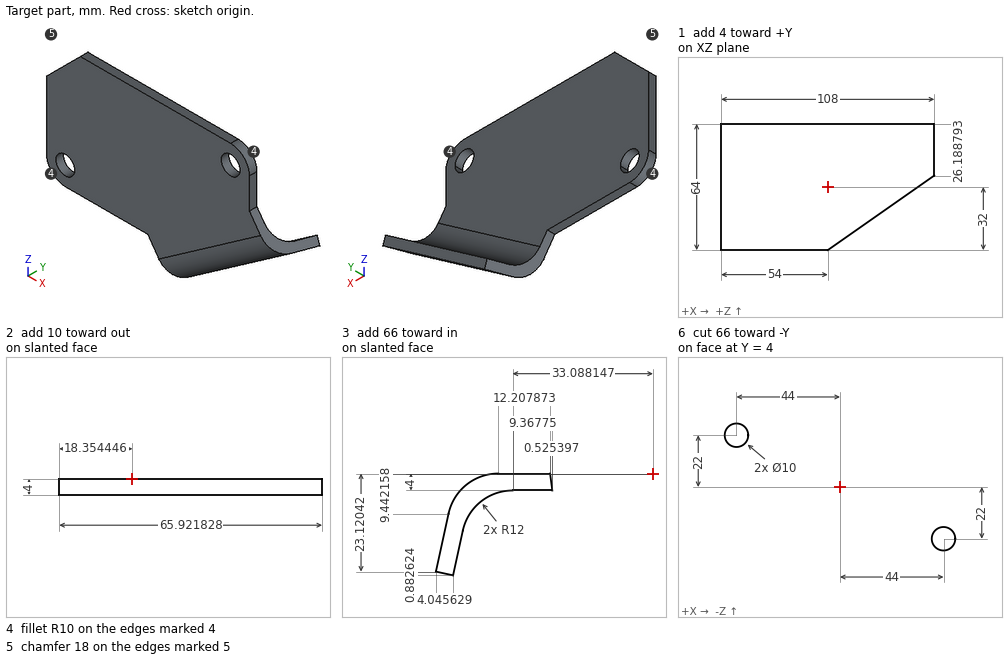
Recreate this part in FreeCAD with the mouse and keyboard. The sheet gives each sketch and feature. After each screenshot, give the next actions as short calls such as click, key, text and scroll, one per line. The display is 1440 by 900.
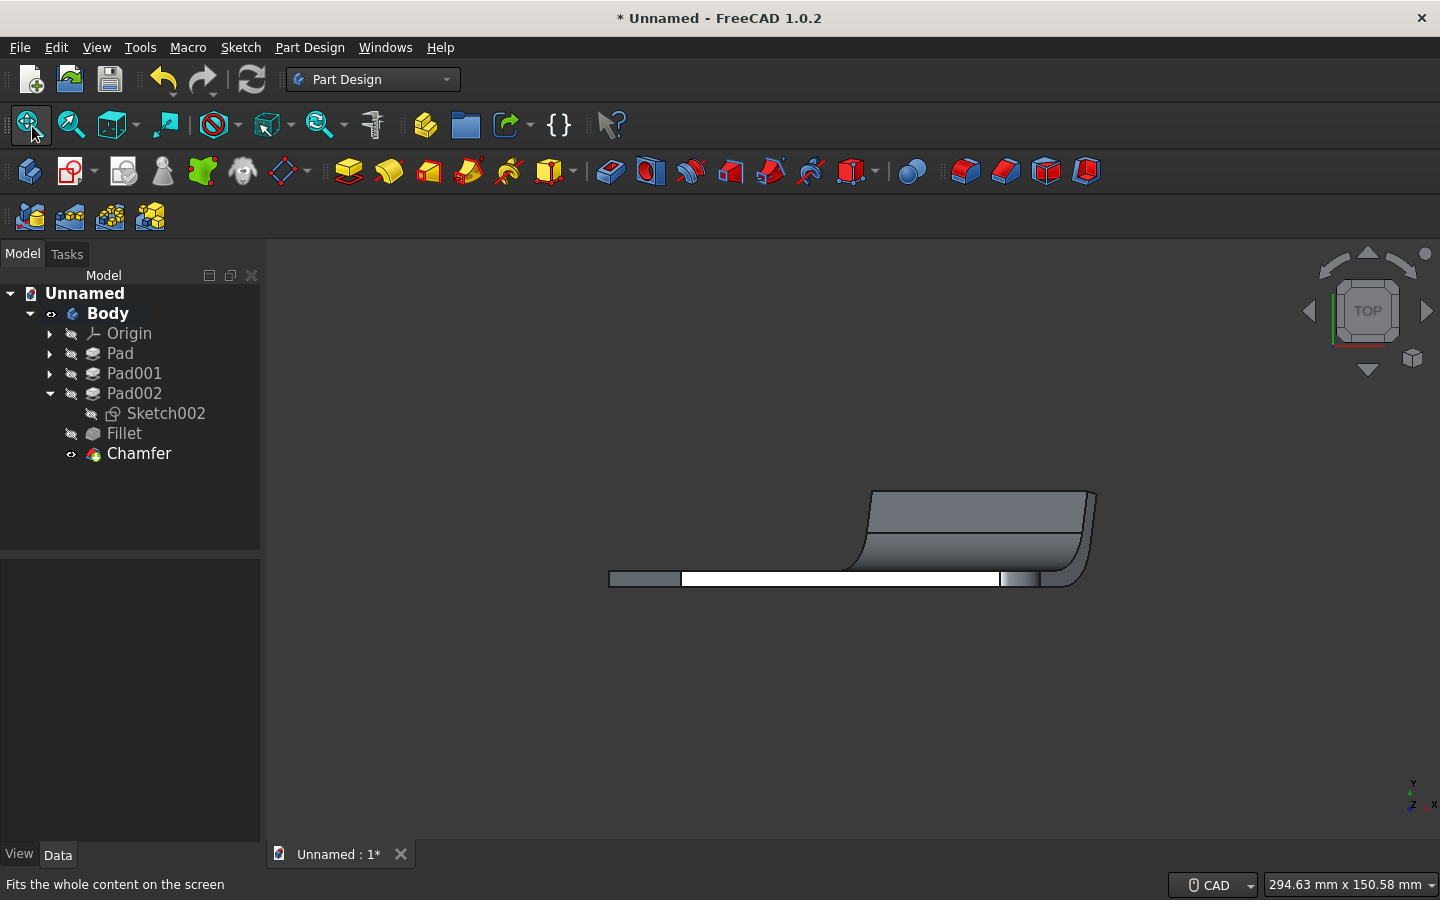
key(4)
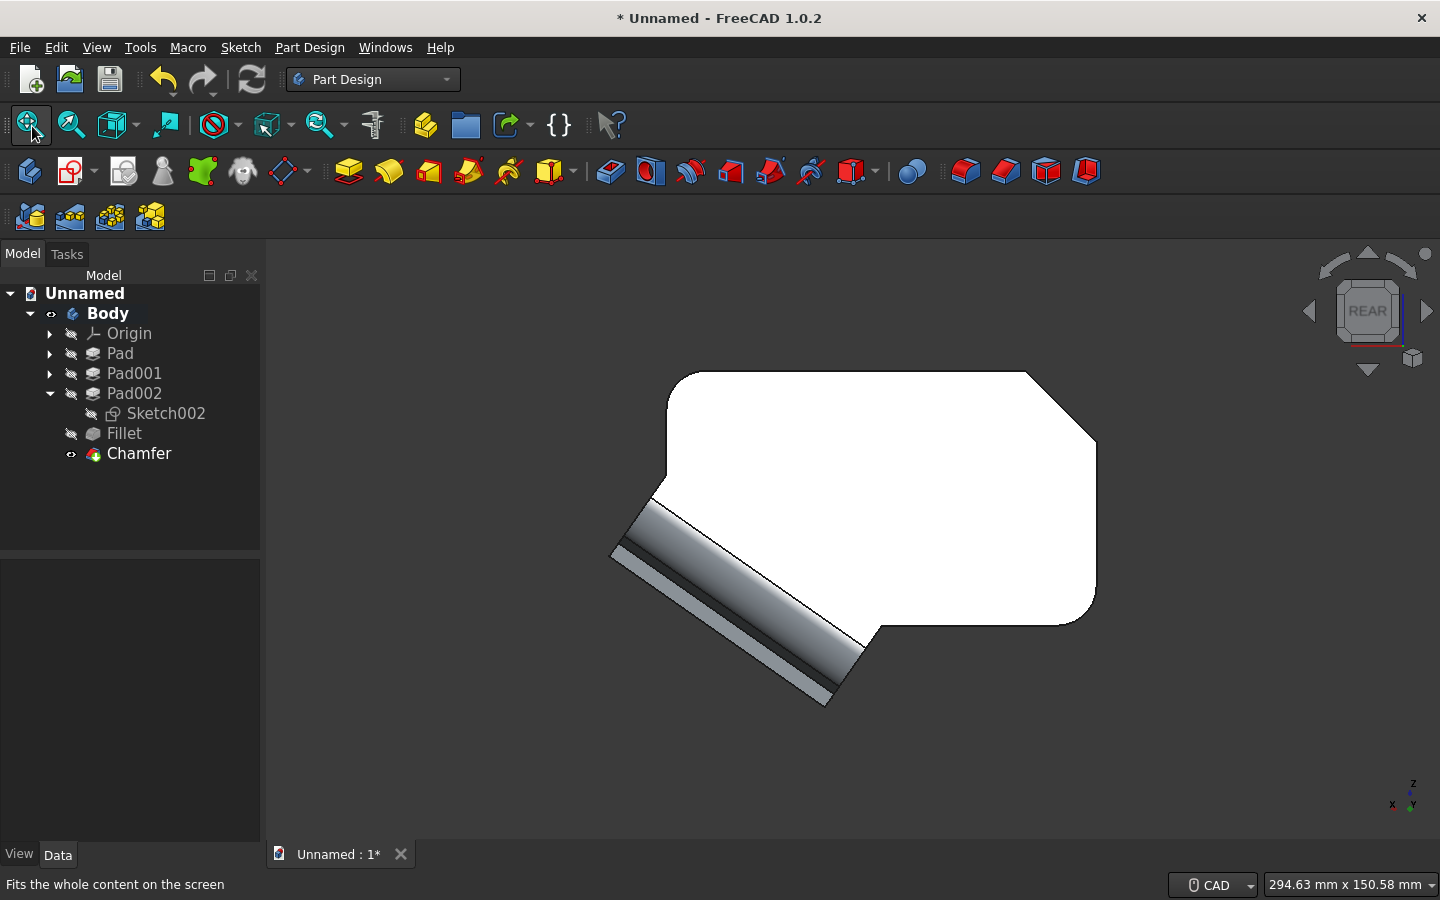
click(874, 509)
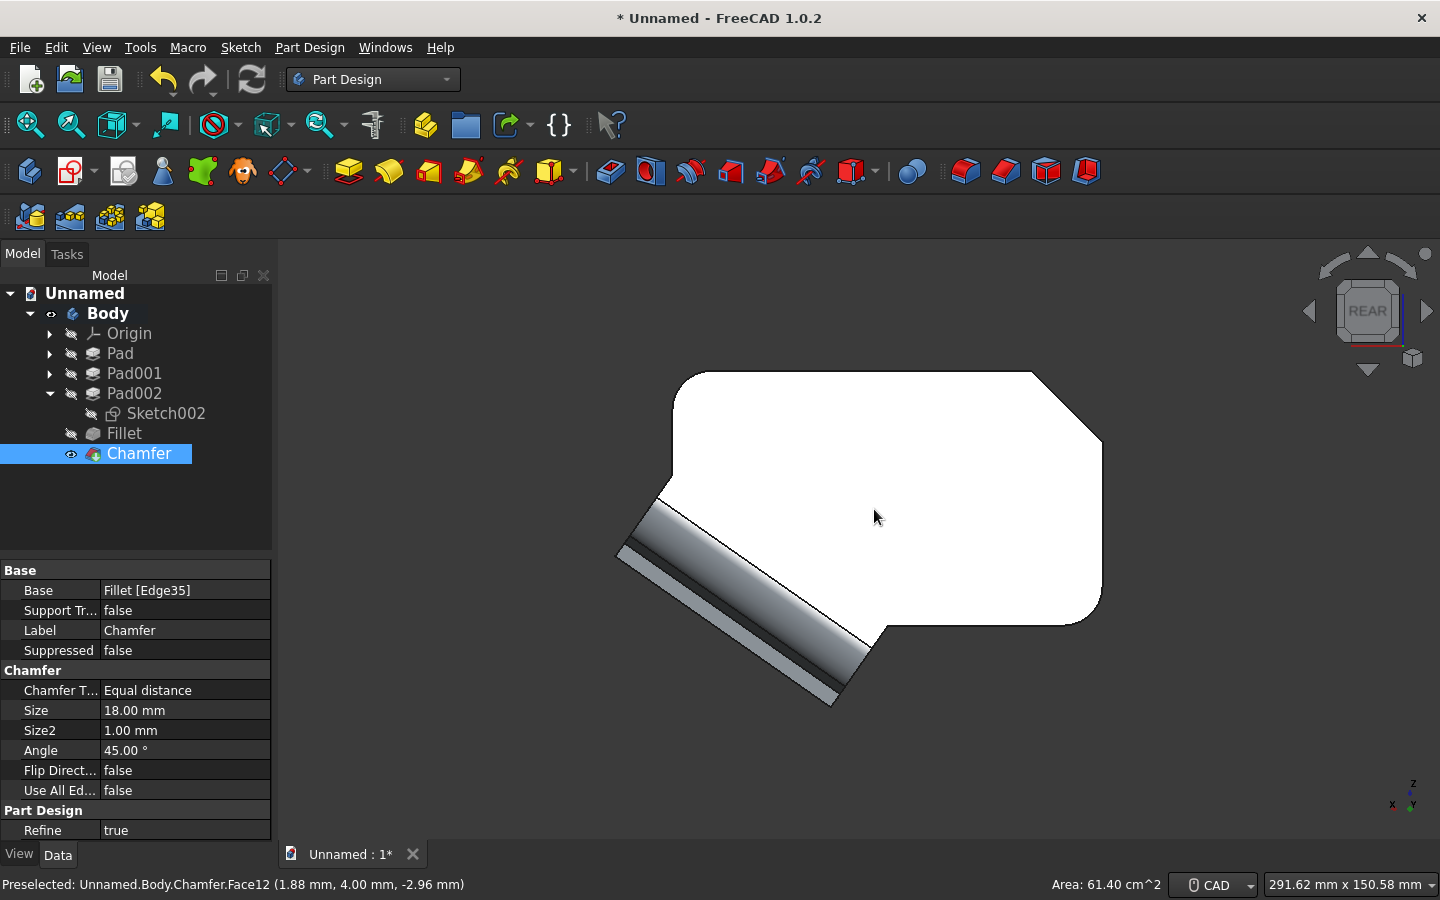
click(70, 172)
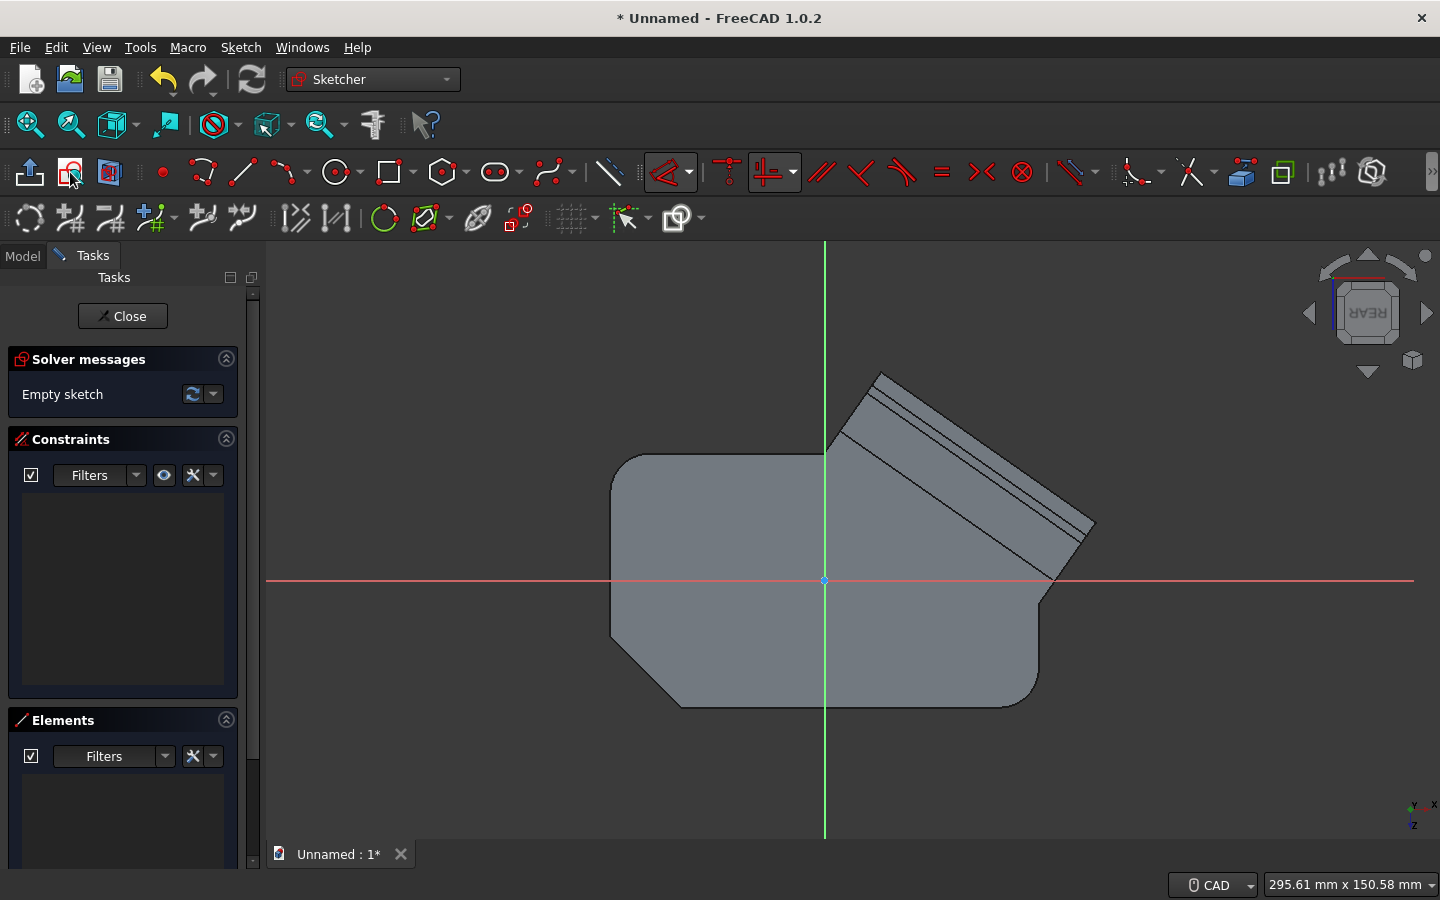
scroll(873, 630, up, 3)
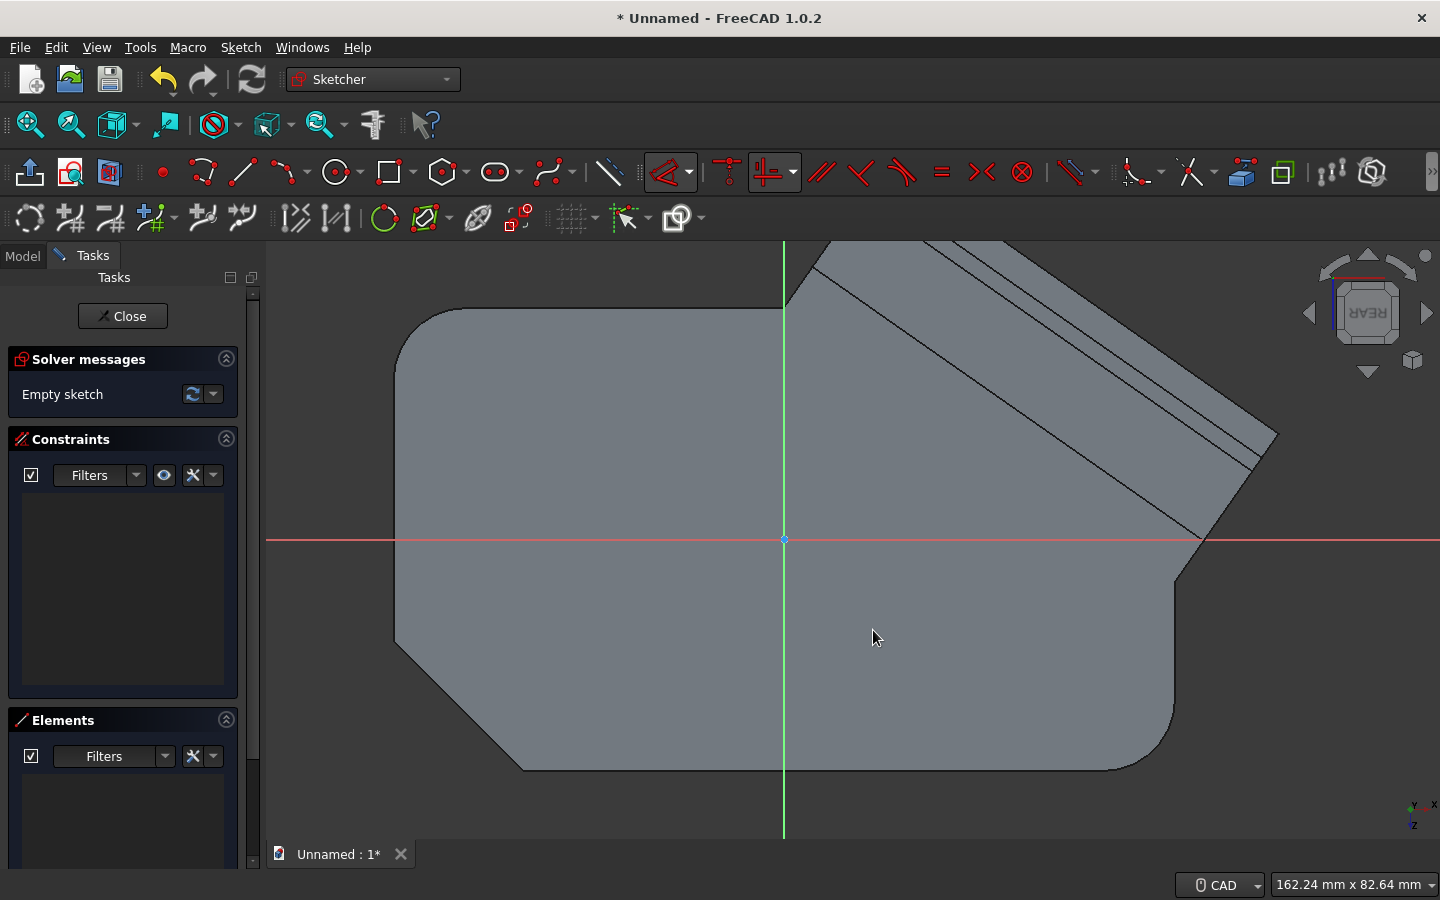
key(g)
key(c)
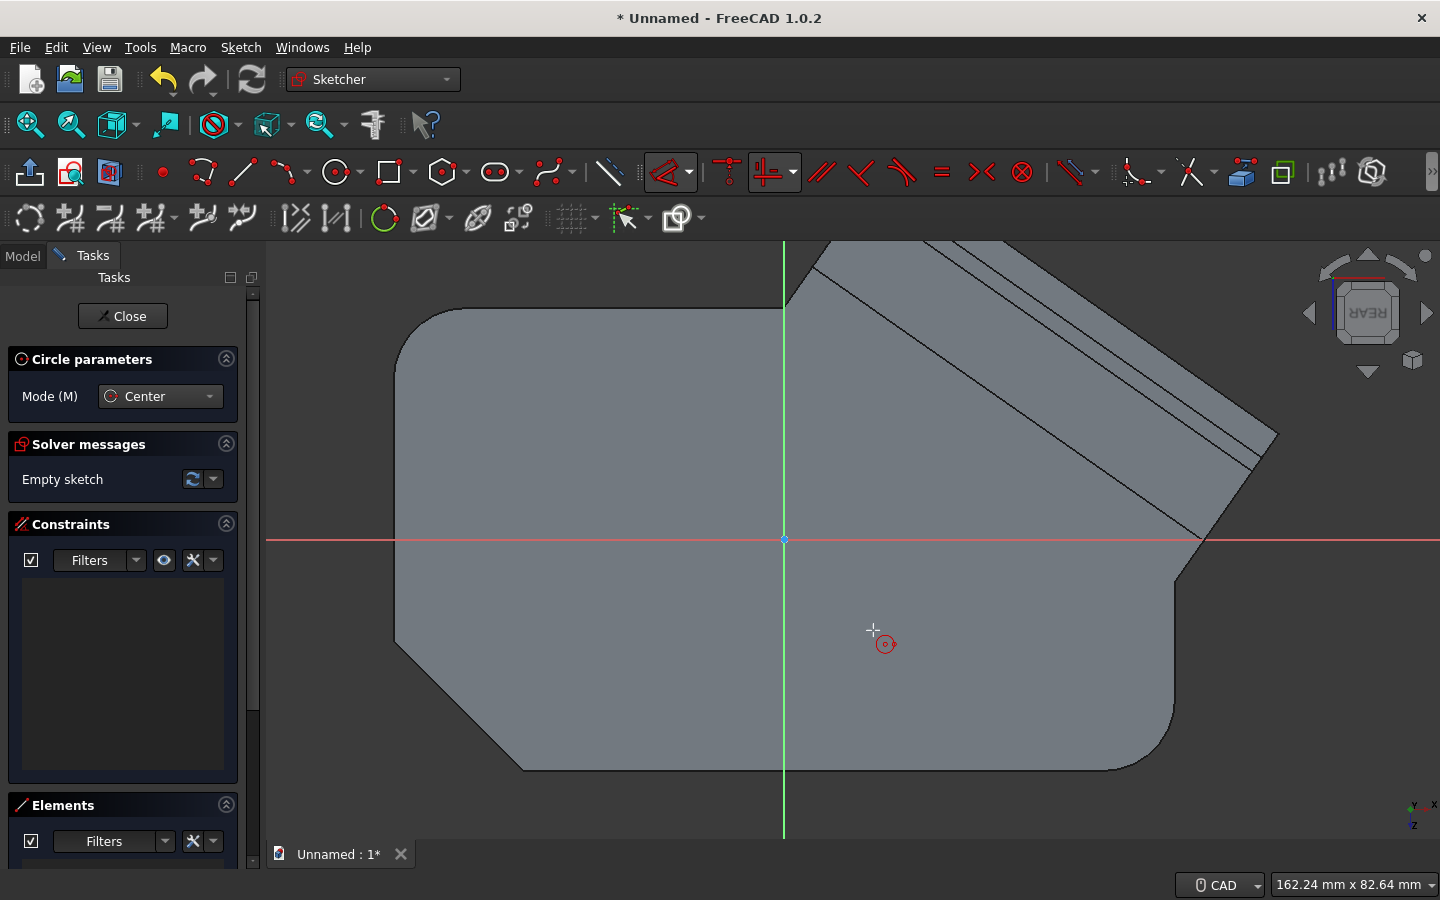
click(466, 380)
click(492, 355)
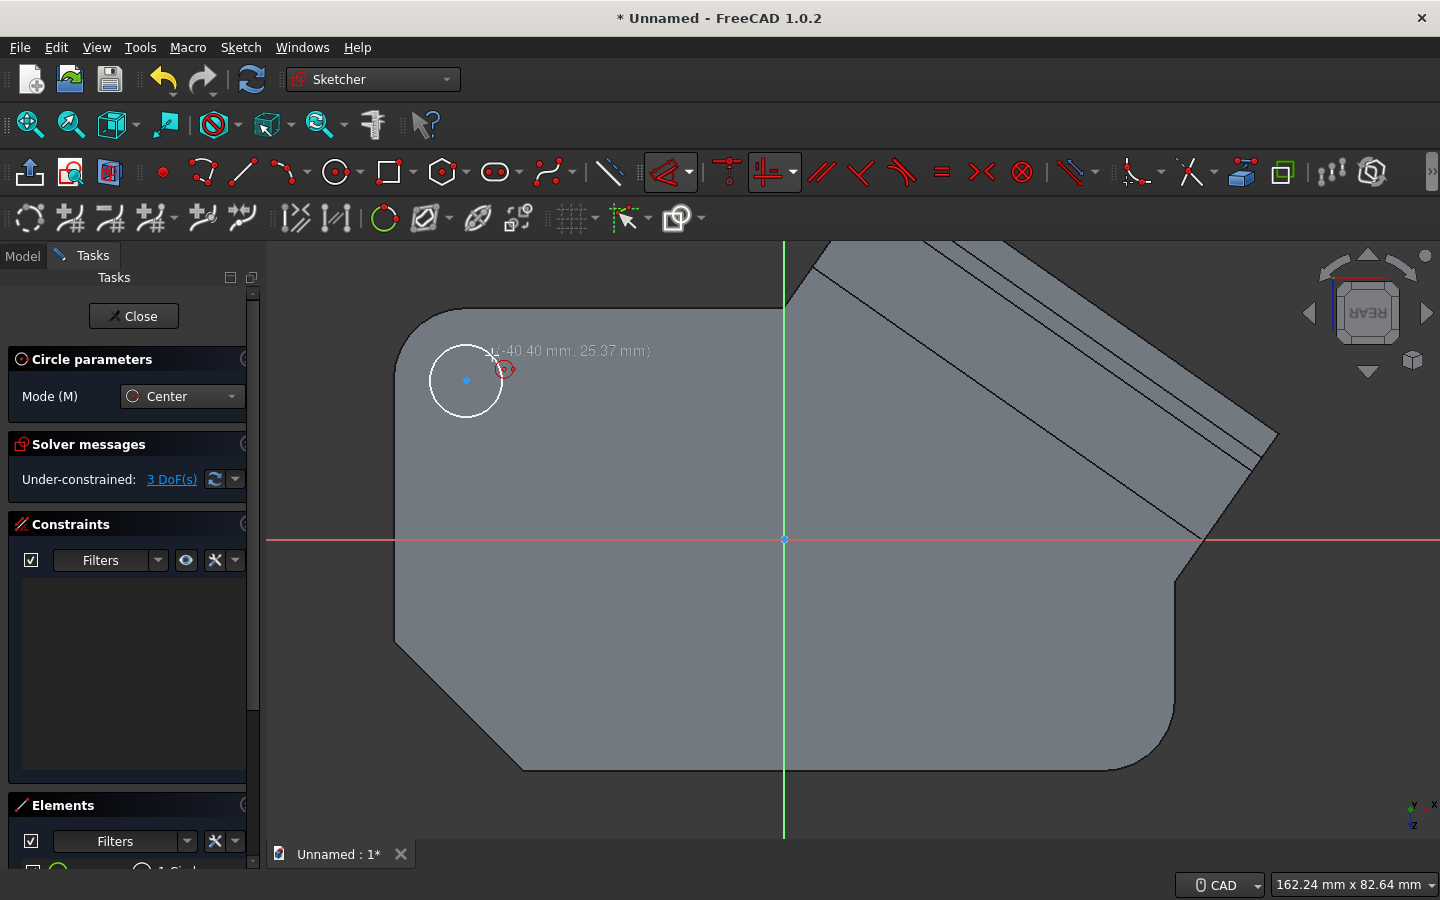
click(1103, 699)
click(1128, 673)
key(Escape)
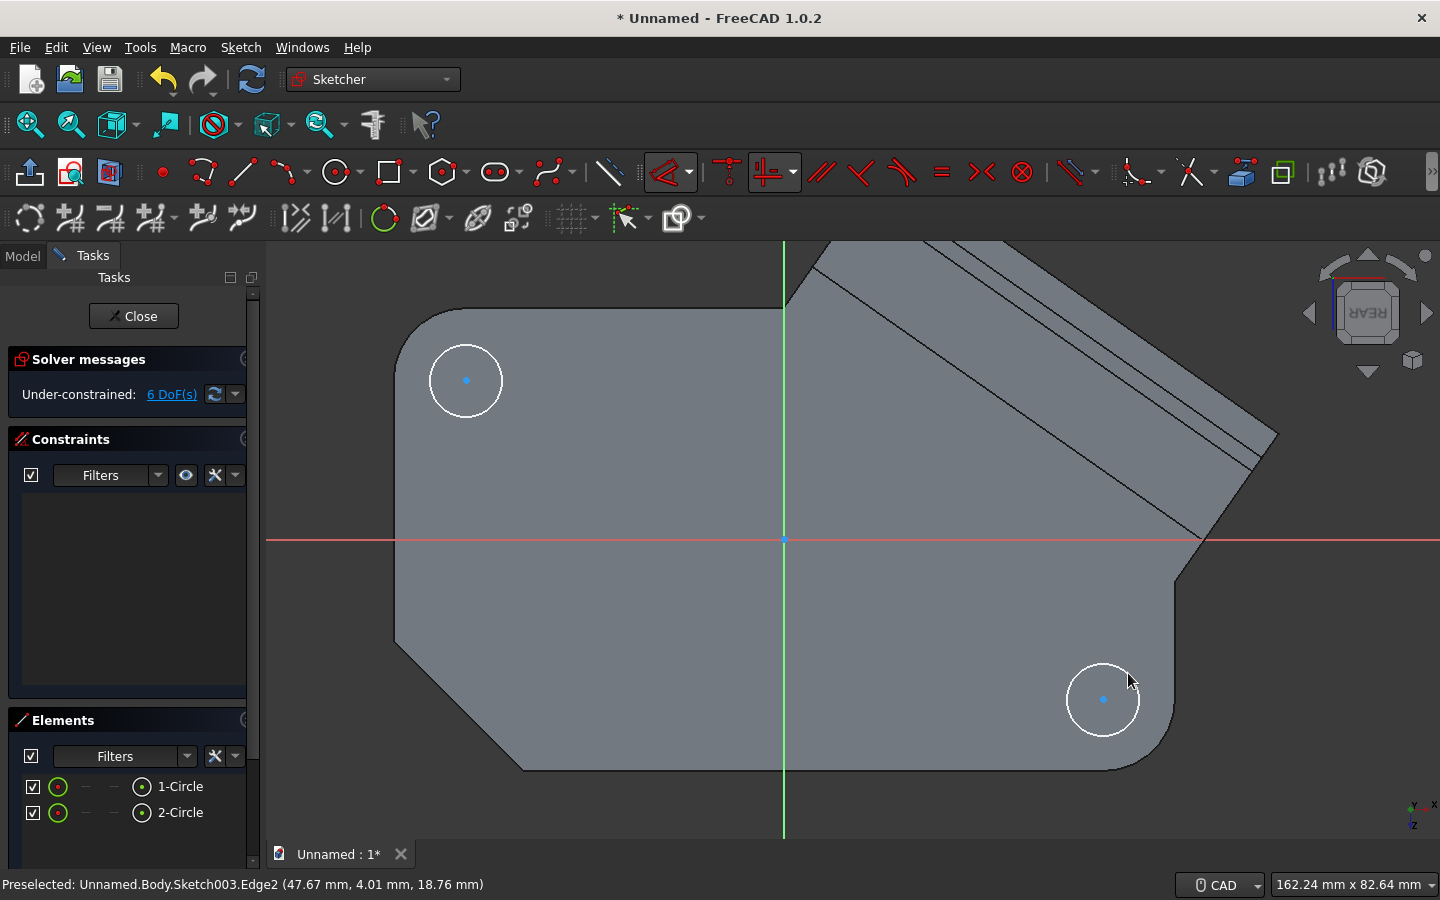
click(491, 355)